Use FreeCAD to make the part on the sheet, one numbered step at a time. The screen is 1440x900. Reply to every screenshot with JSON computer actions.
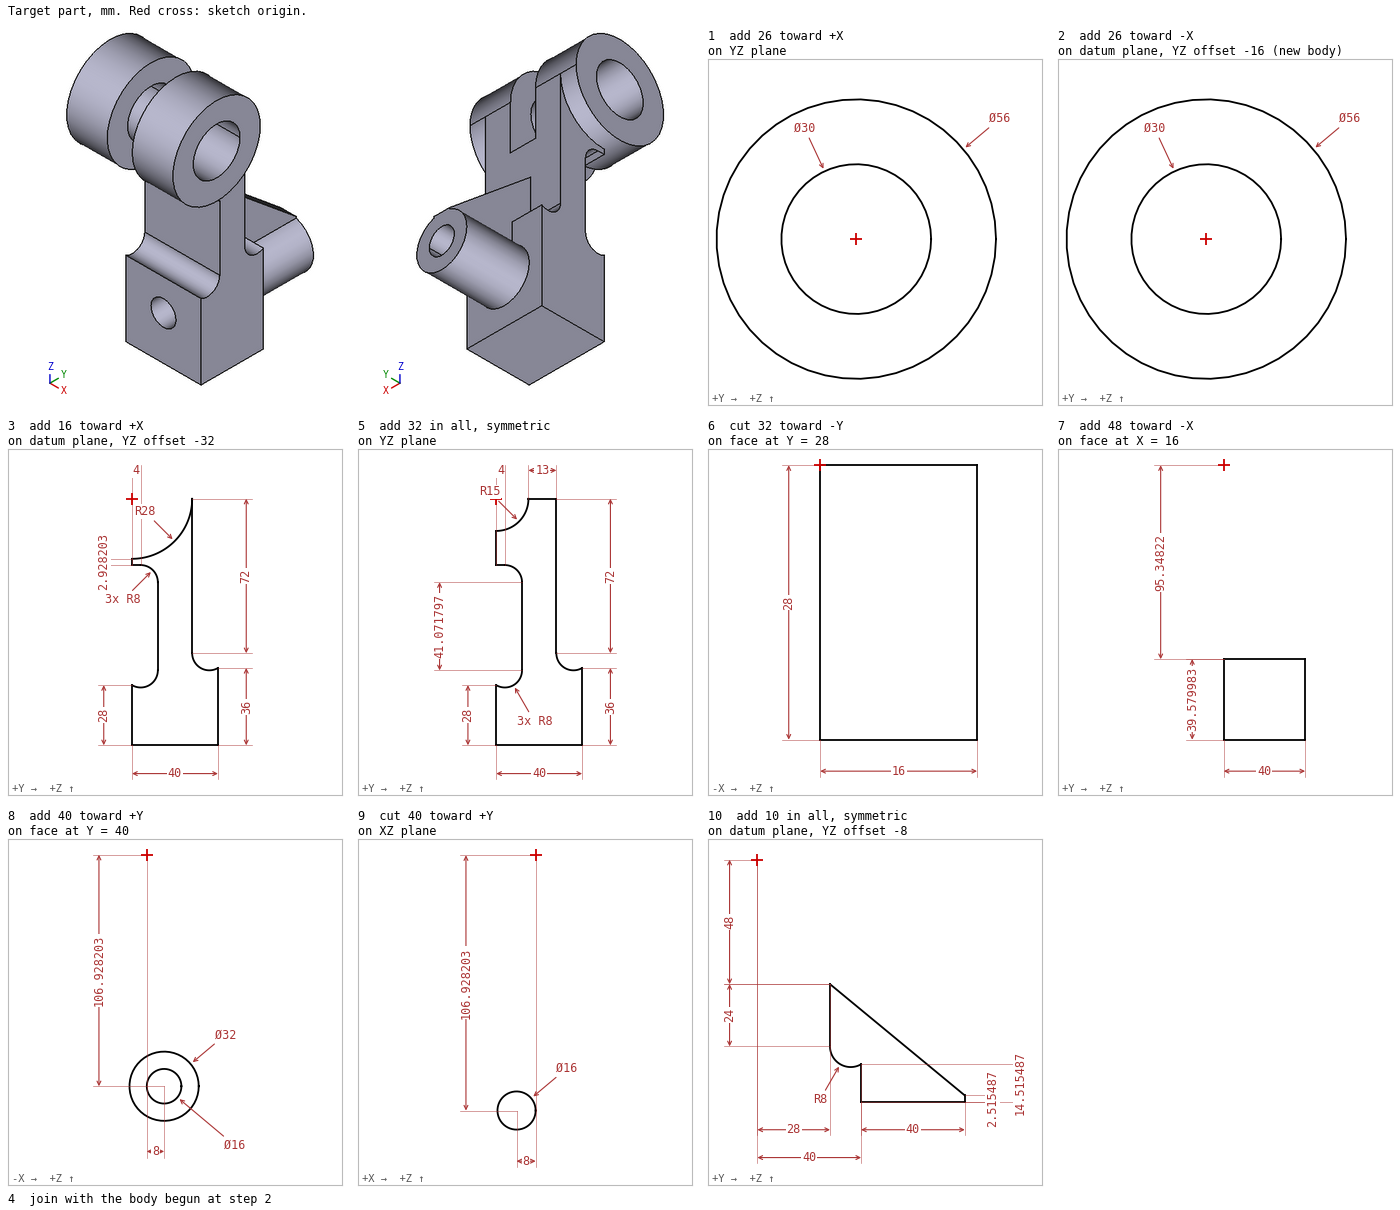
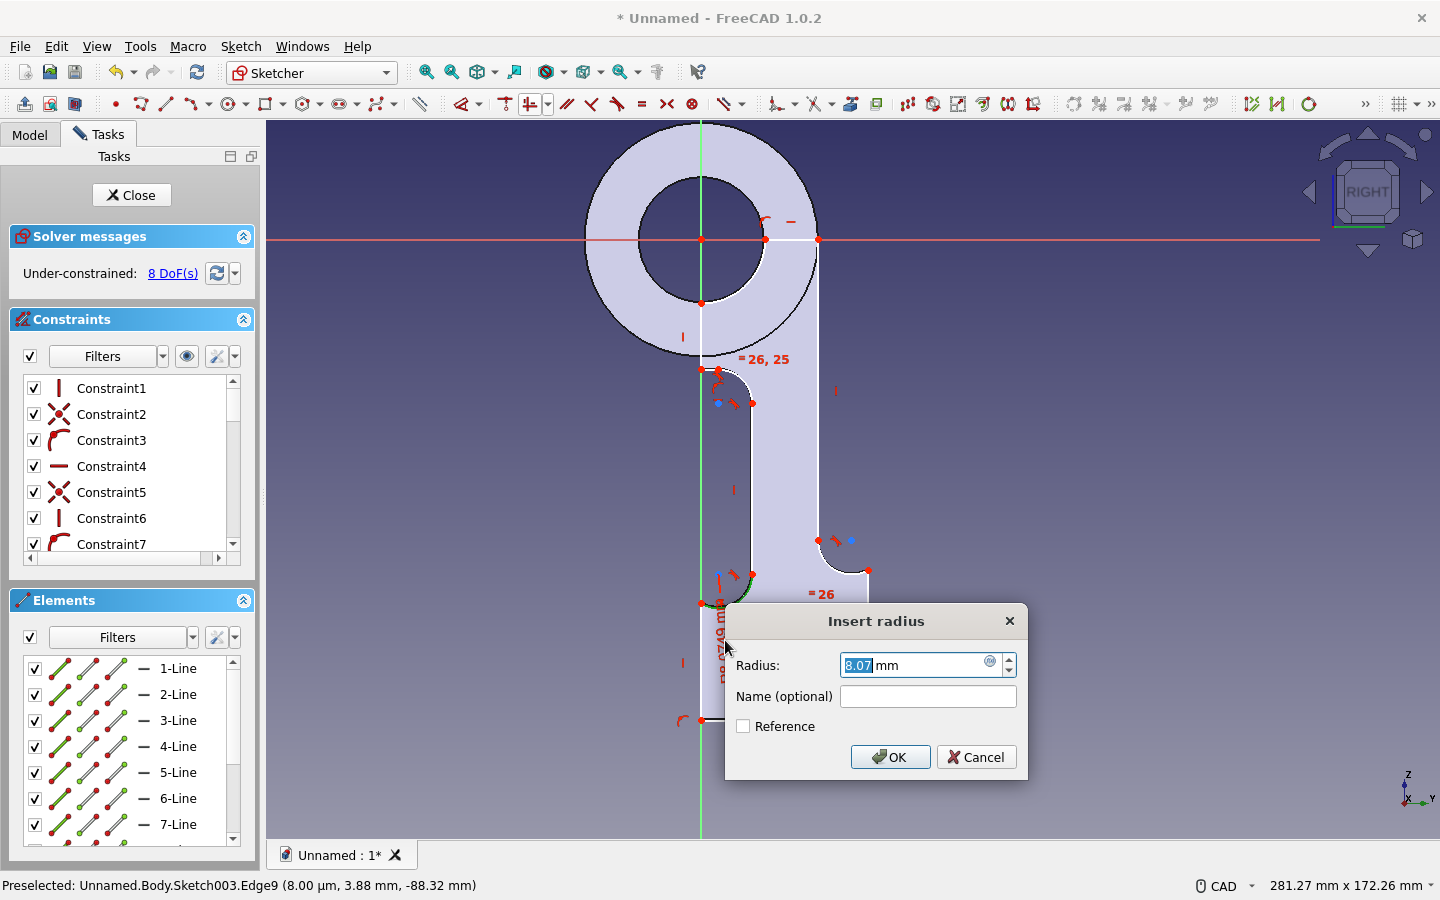
{"action": "type", "text": "8"}
{"action": "key", "text": "Return"}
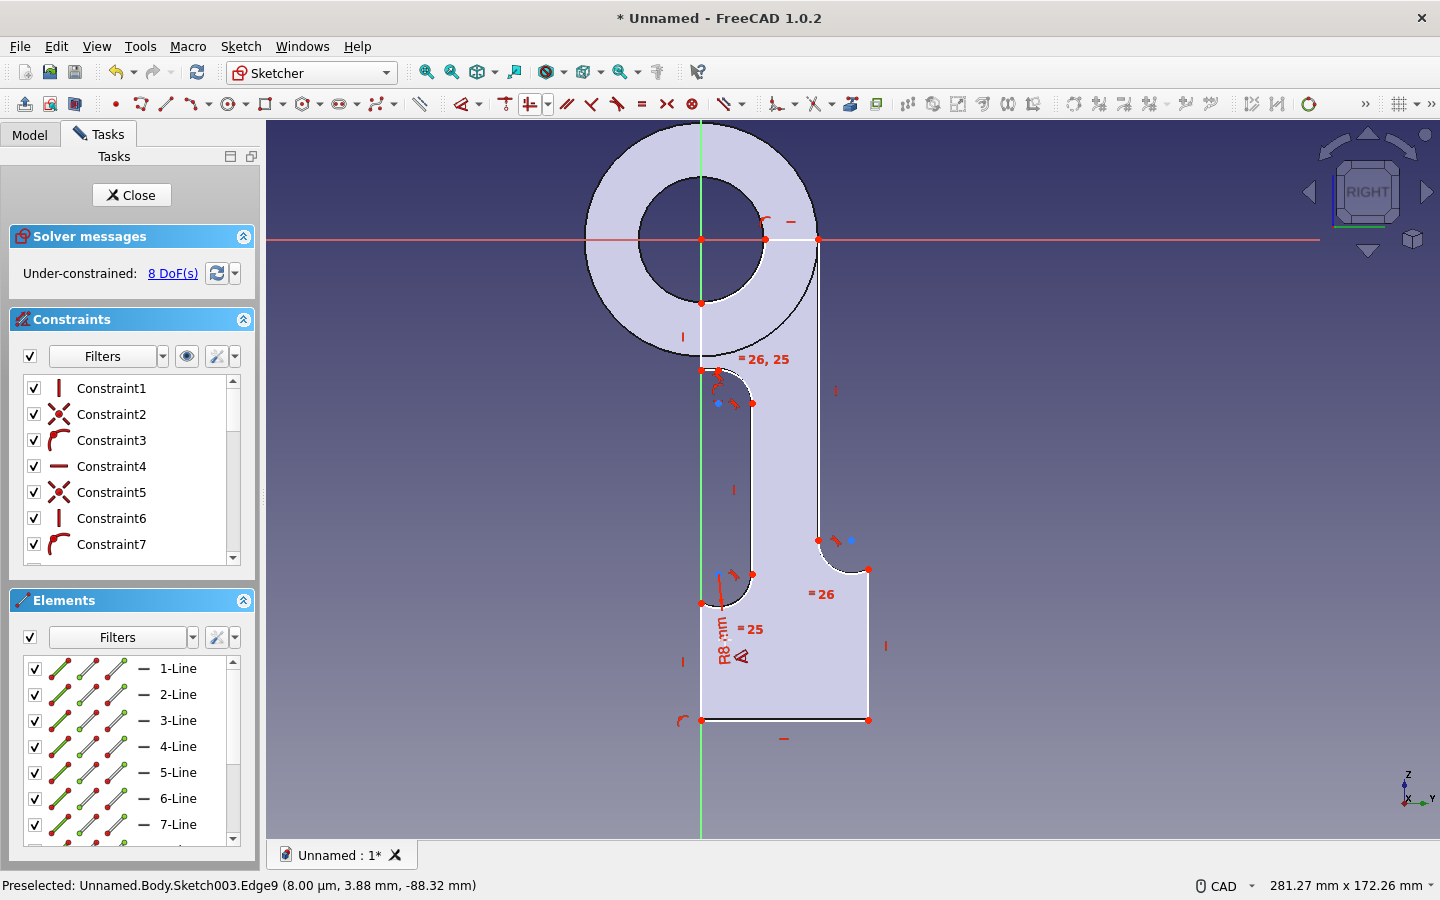
{"action": "left_click", "coordinate": [730, 297]}
{"action": "left_click", "coordinate": [744, 326]}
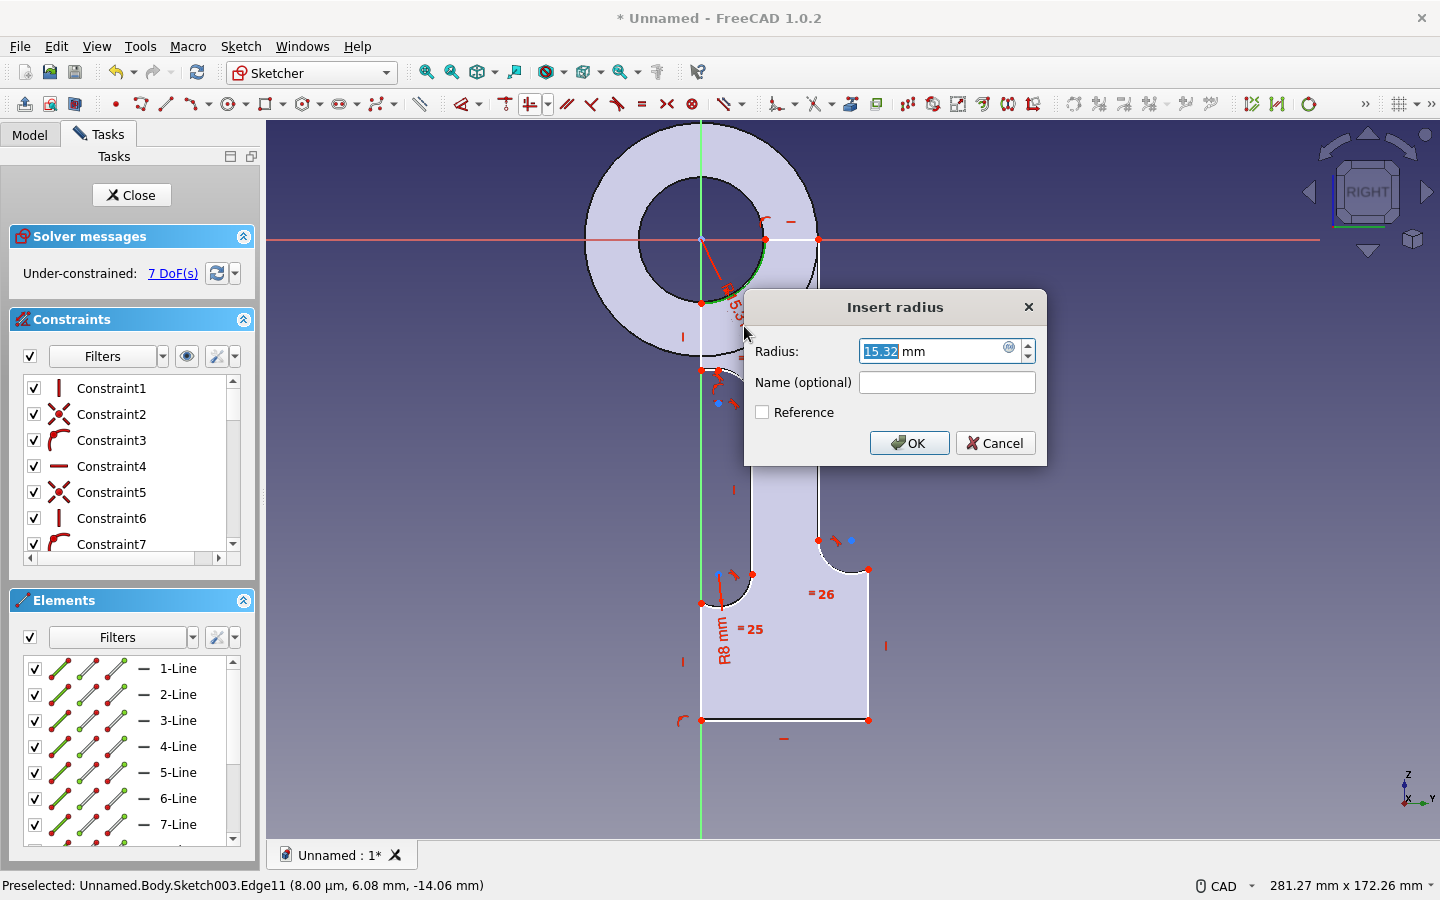
{"action": "type", "text": "15"}
{"action": "key", "text": "Return"}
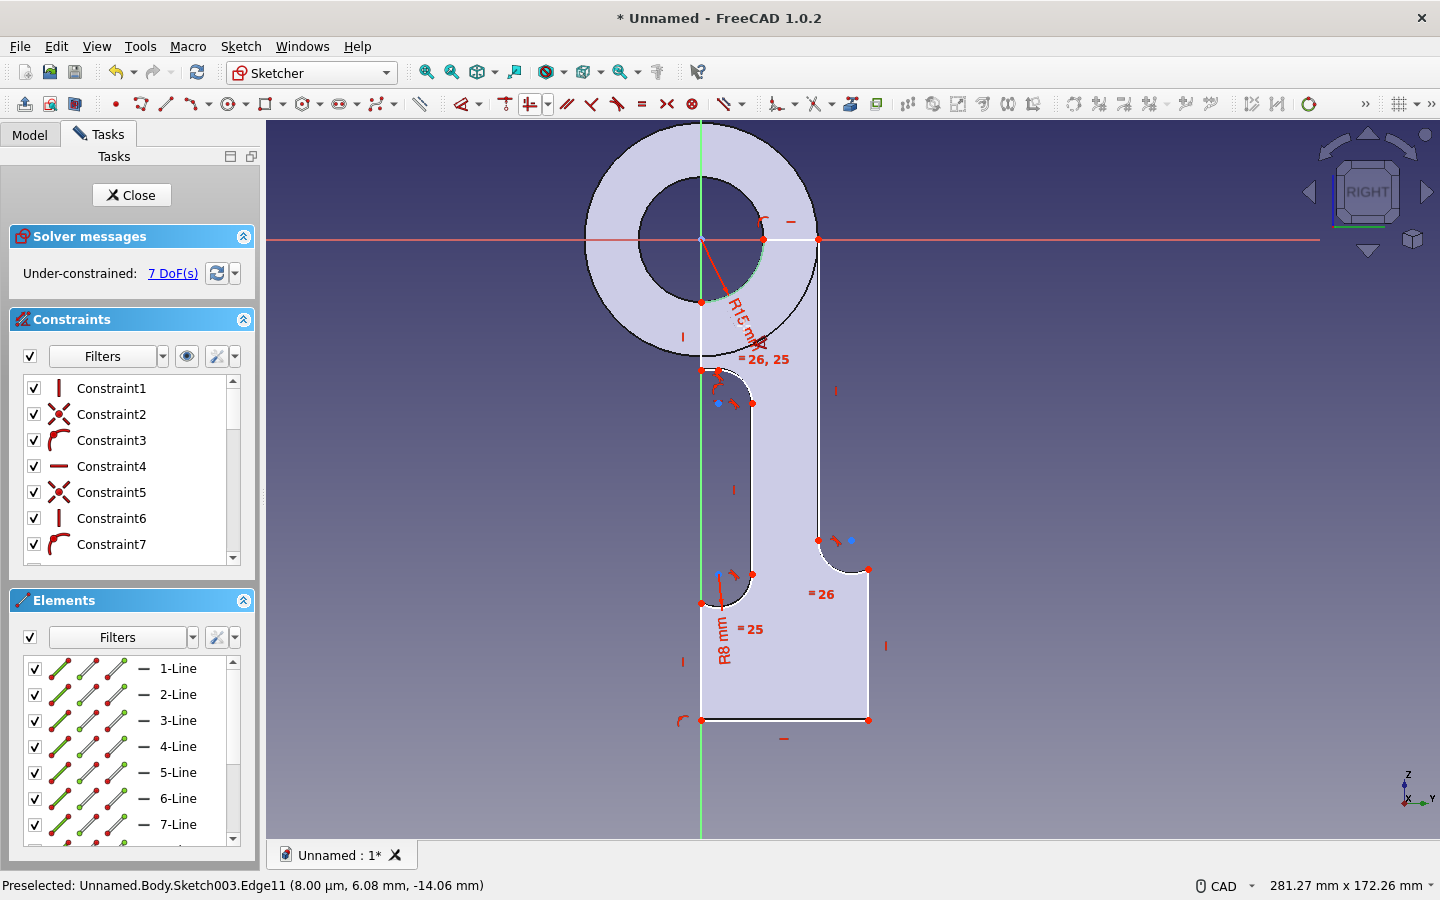
{"action": "scroll", "coordinate": [710, 370], "scroll_direction": "up", "scroll_amount": 5}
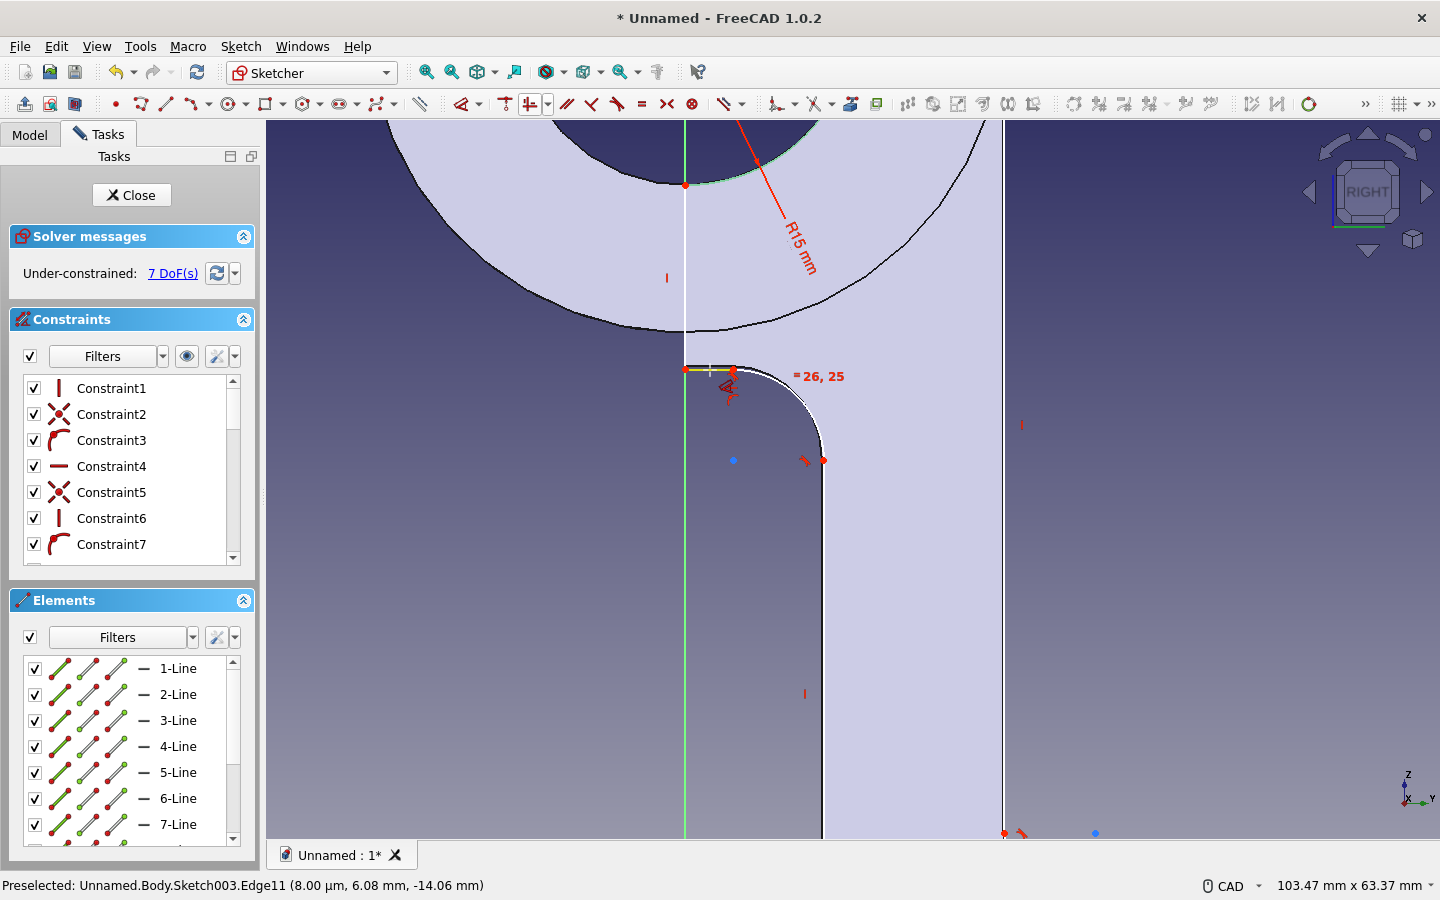
{"action": "left_click", "coordinate": [709, 370]}
{"action": "left_click", "coordinate": [709, 336]}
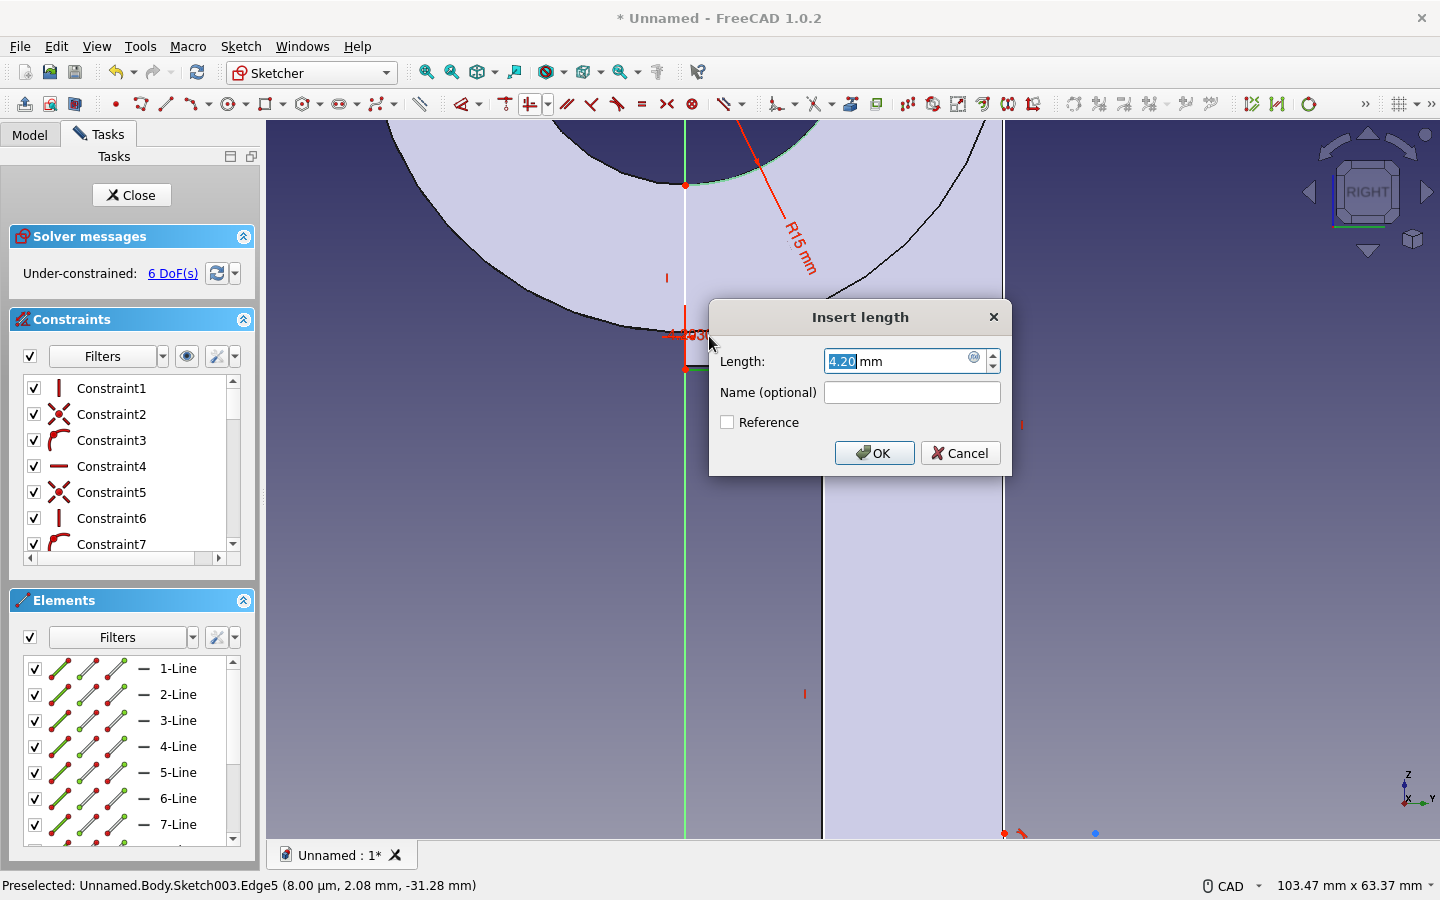
{"action": "type", "text": "4"}
{"action": "key", "text": "Return"}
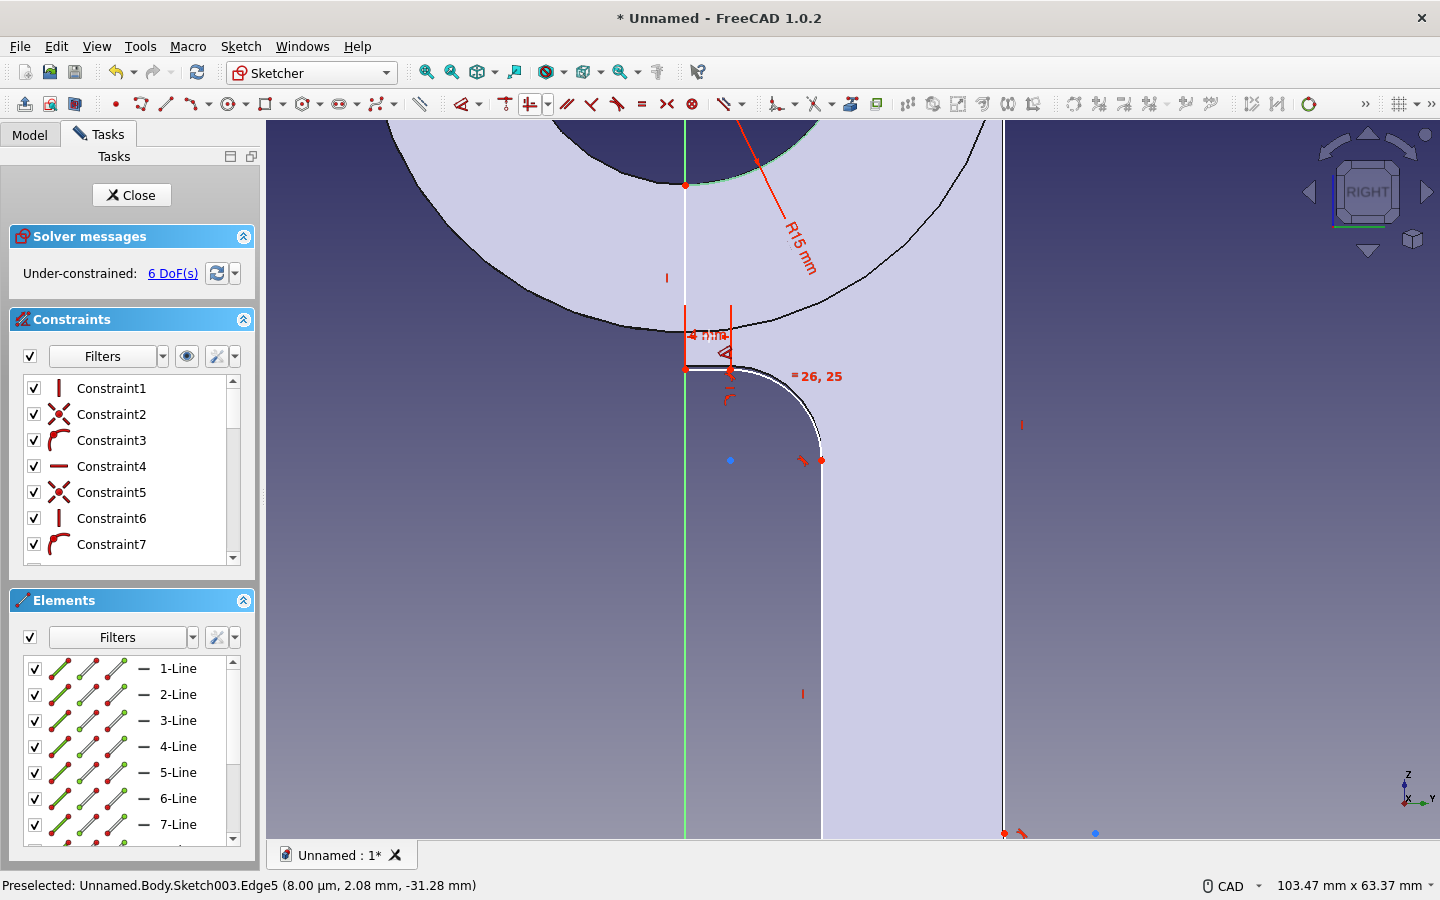
{"action": "scroll", "coordinate": [710, 370], "scroll_direction": "down", "scroll_amount": 5}